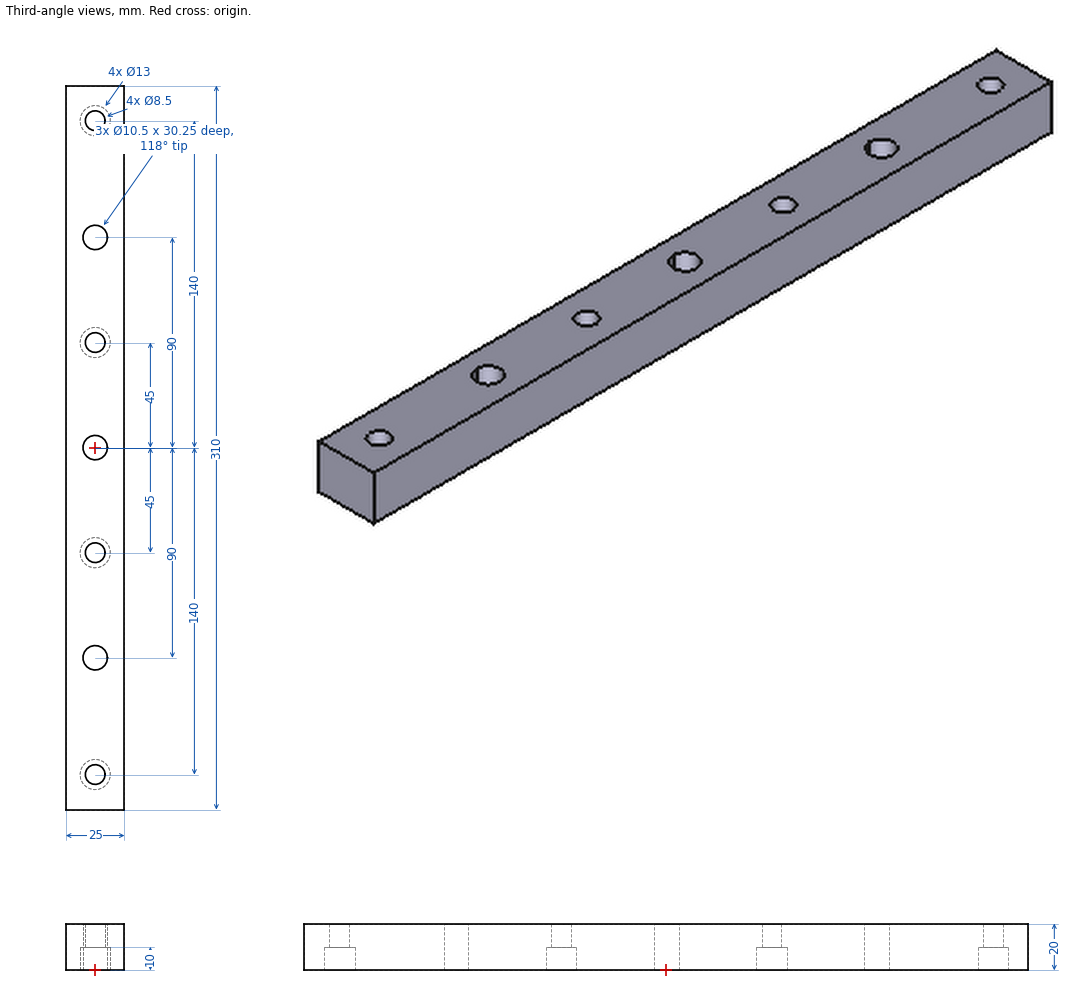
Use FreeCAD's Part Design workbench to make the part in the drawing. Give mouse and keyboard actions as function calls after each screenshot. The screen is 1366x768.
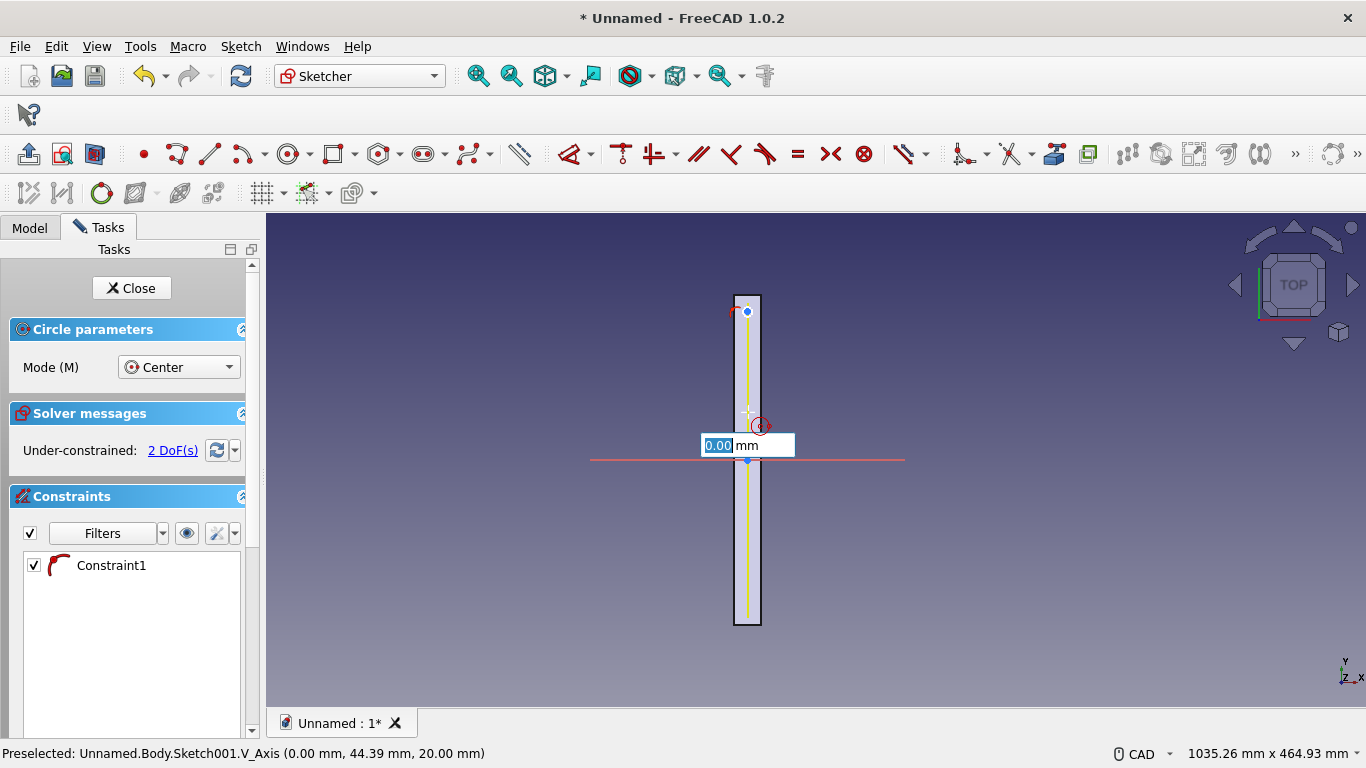
scroll(752, 411, up, 7)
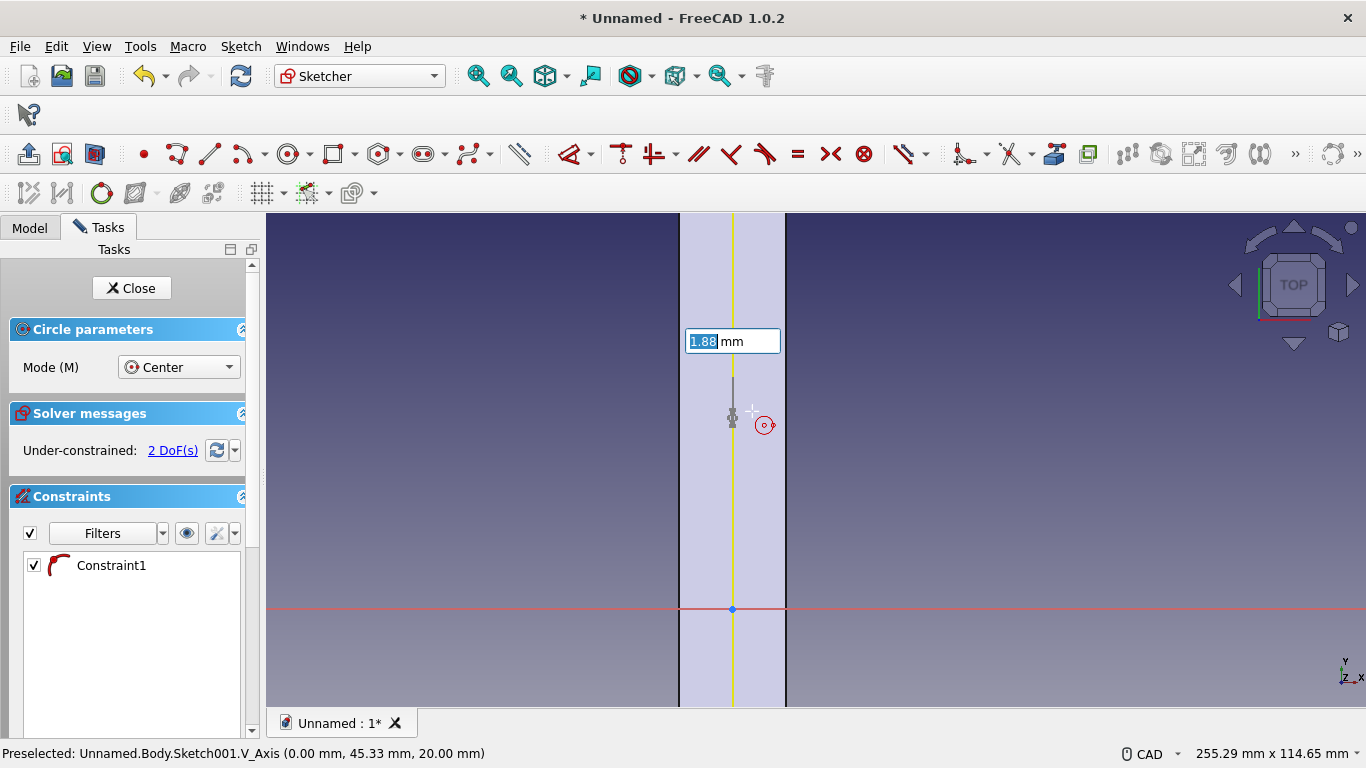
click(750, 409)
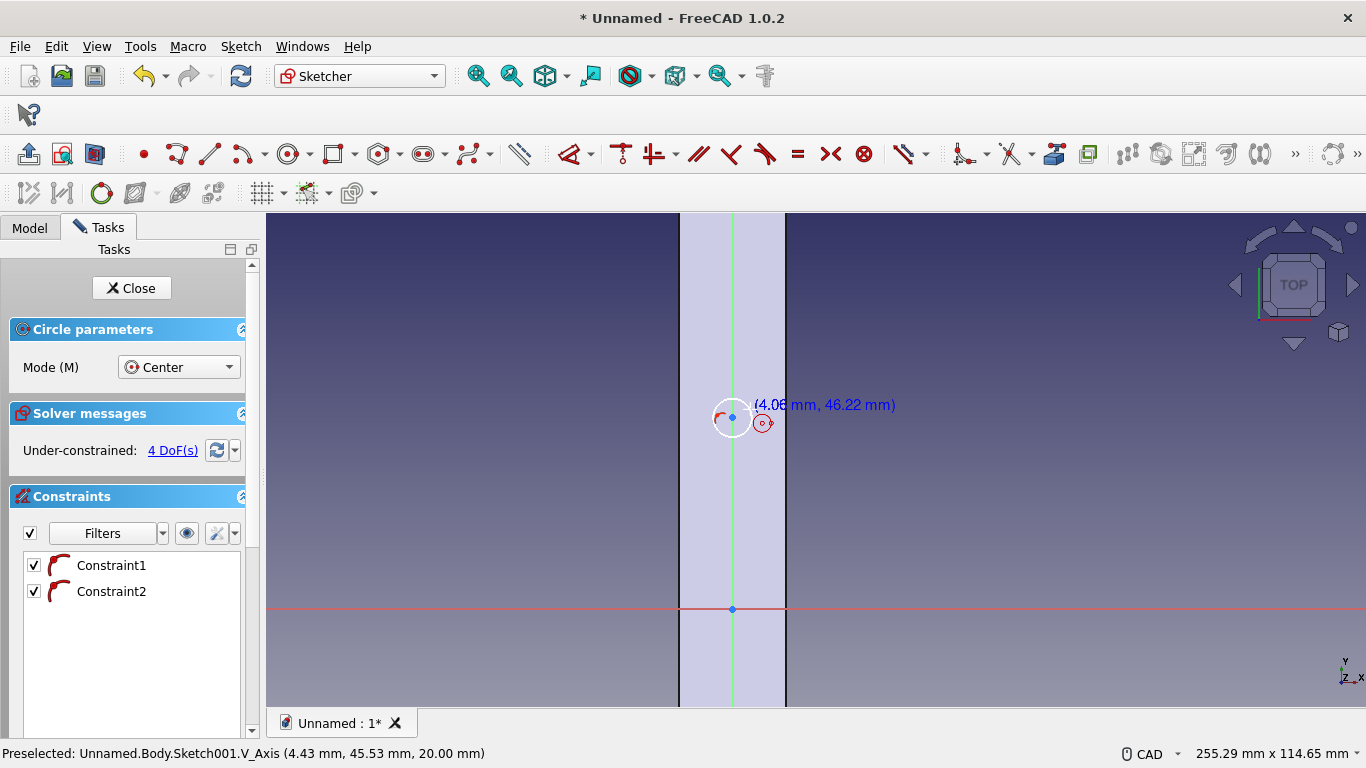
scroll(752, 411, down, 7)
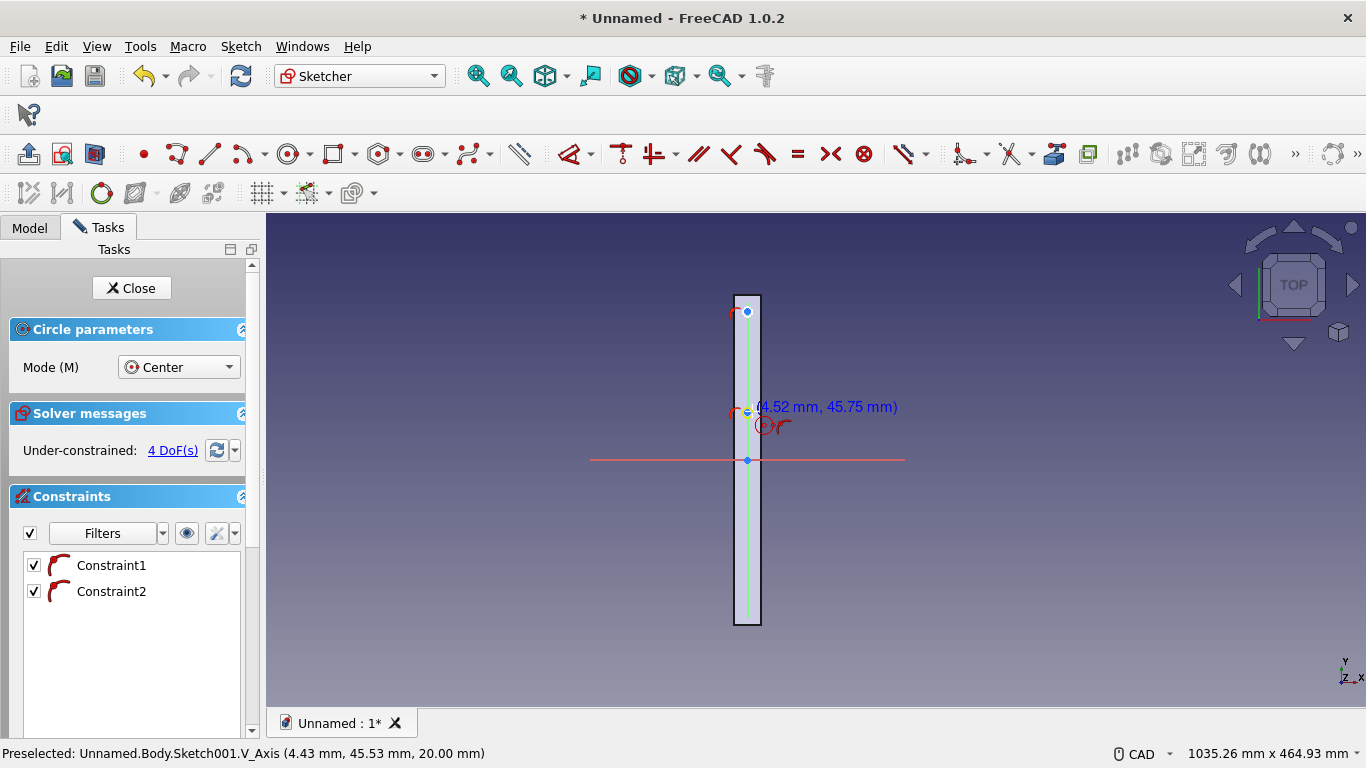
scroll(748, 508, up, 9)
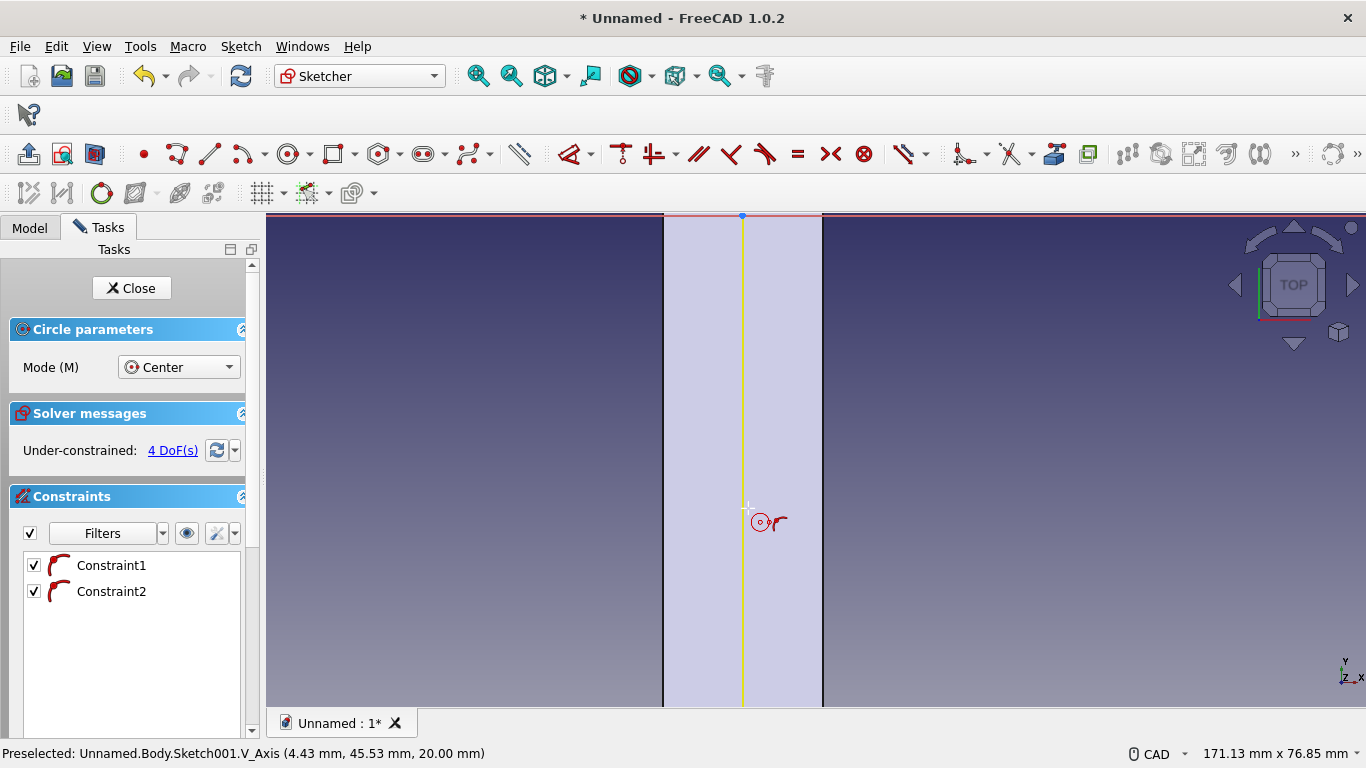
scroll(748, 508, down, 9)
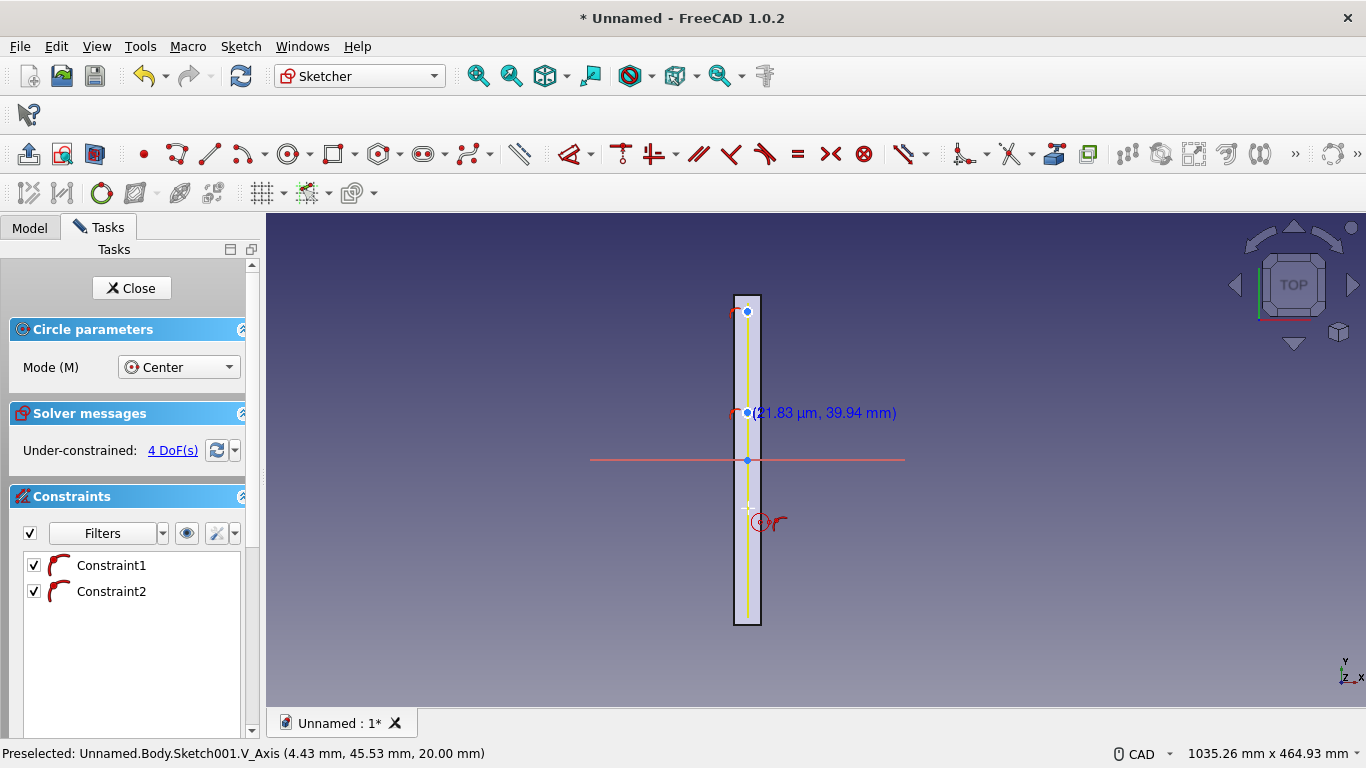
click(748, 508)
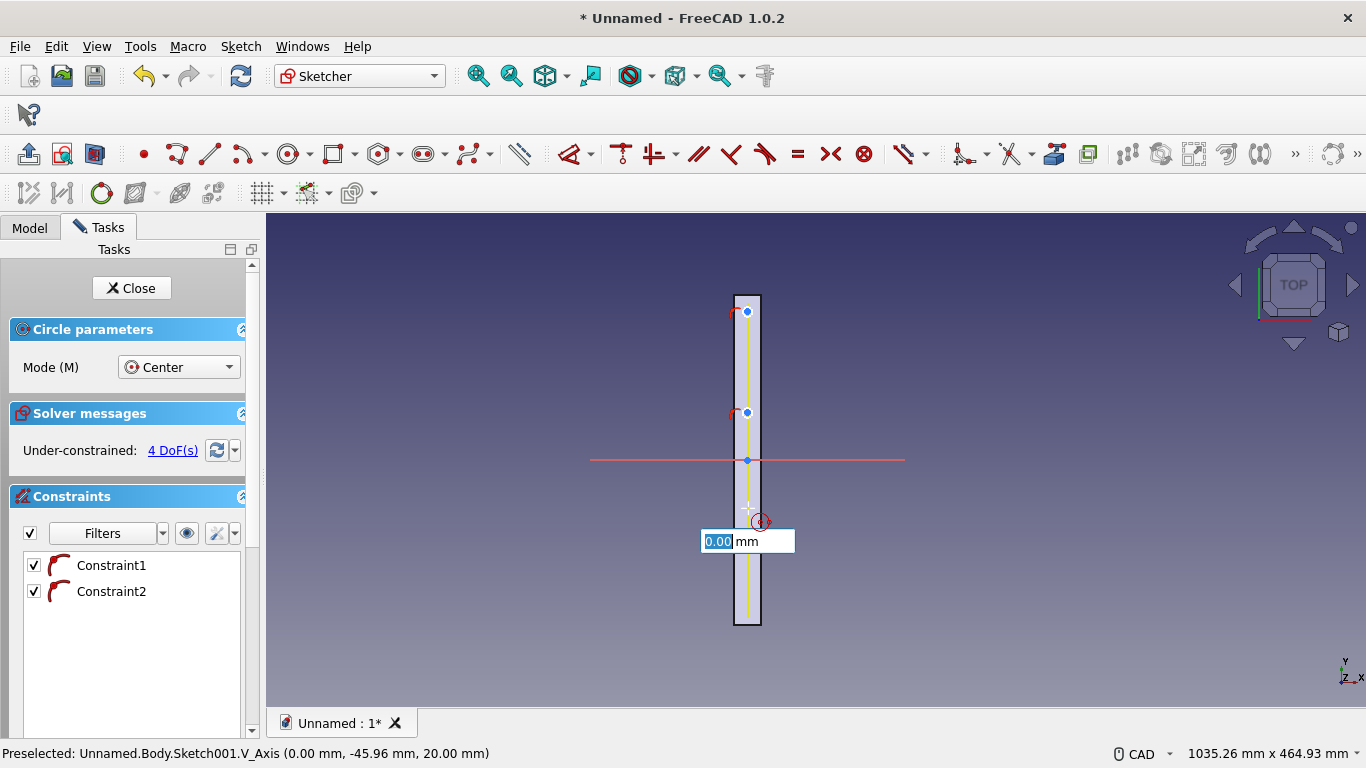
scroll(752, 506, up, 7)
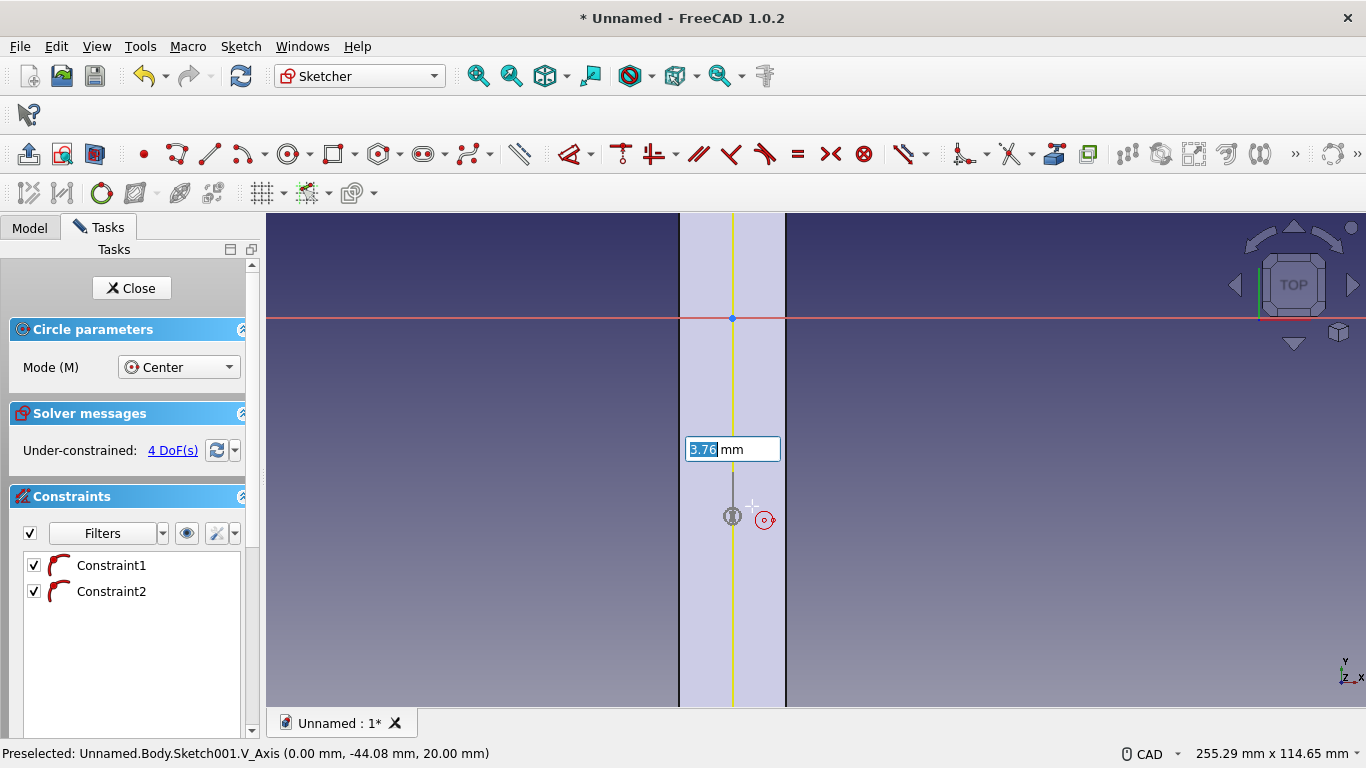
click(750, 506)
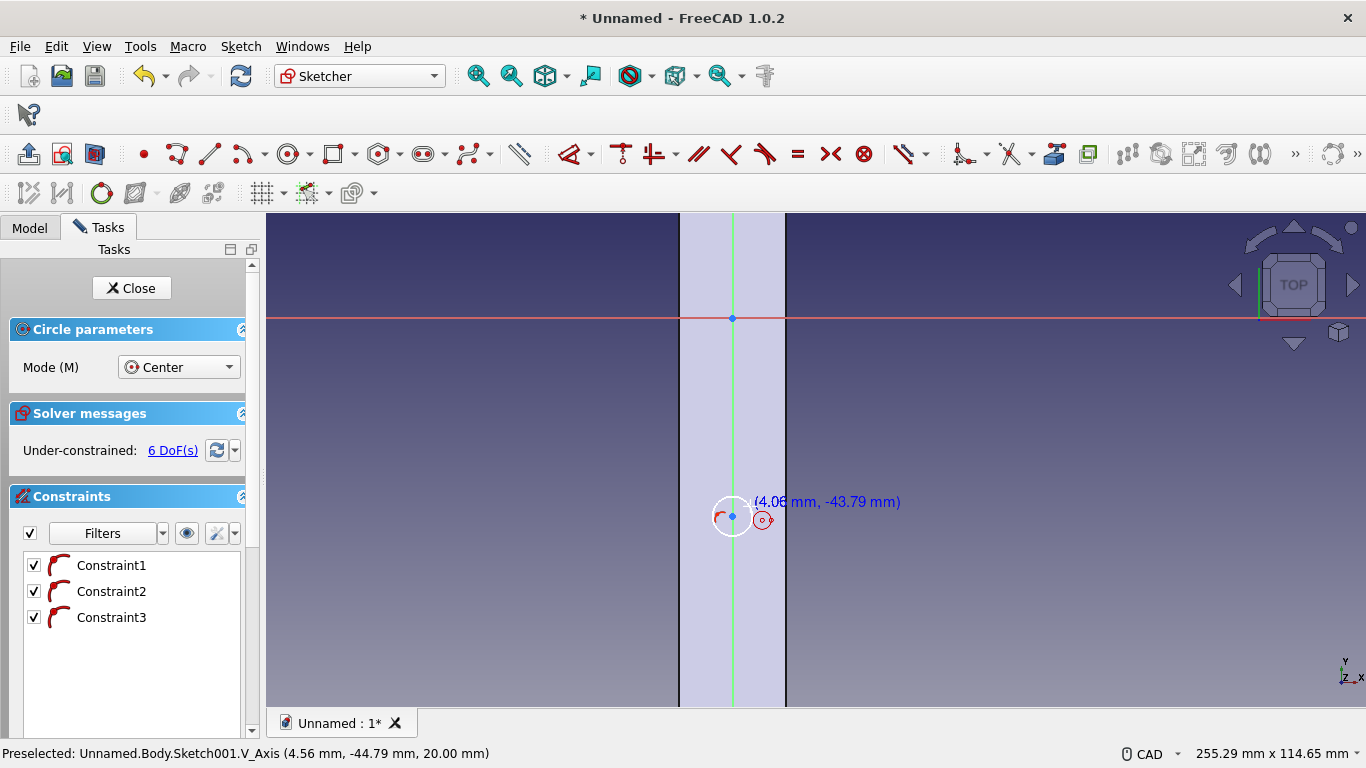
scroll(752, 506, down, 7)